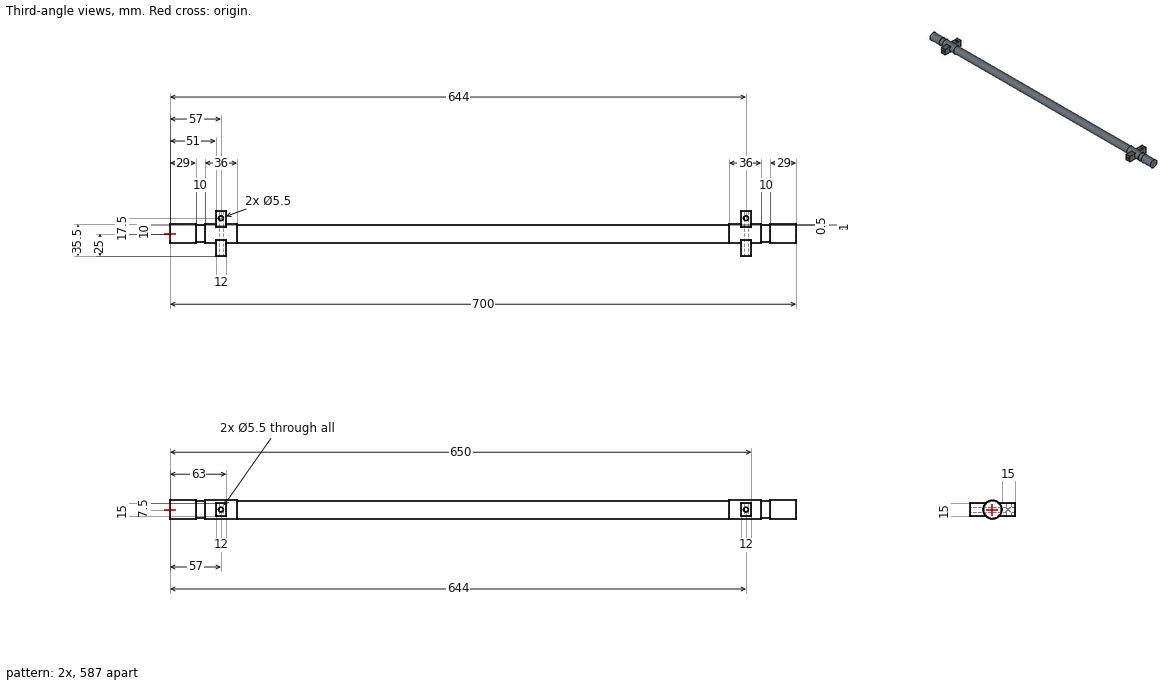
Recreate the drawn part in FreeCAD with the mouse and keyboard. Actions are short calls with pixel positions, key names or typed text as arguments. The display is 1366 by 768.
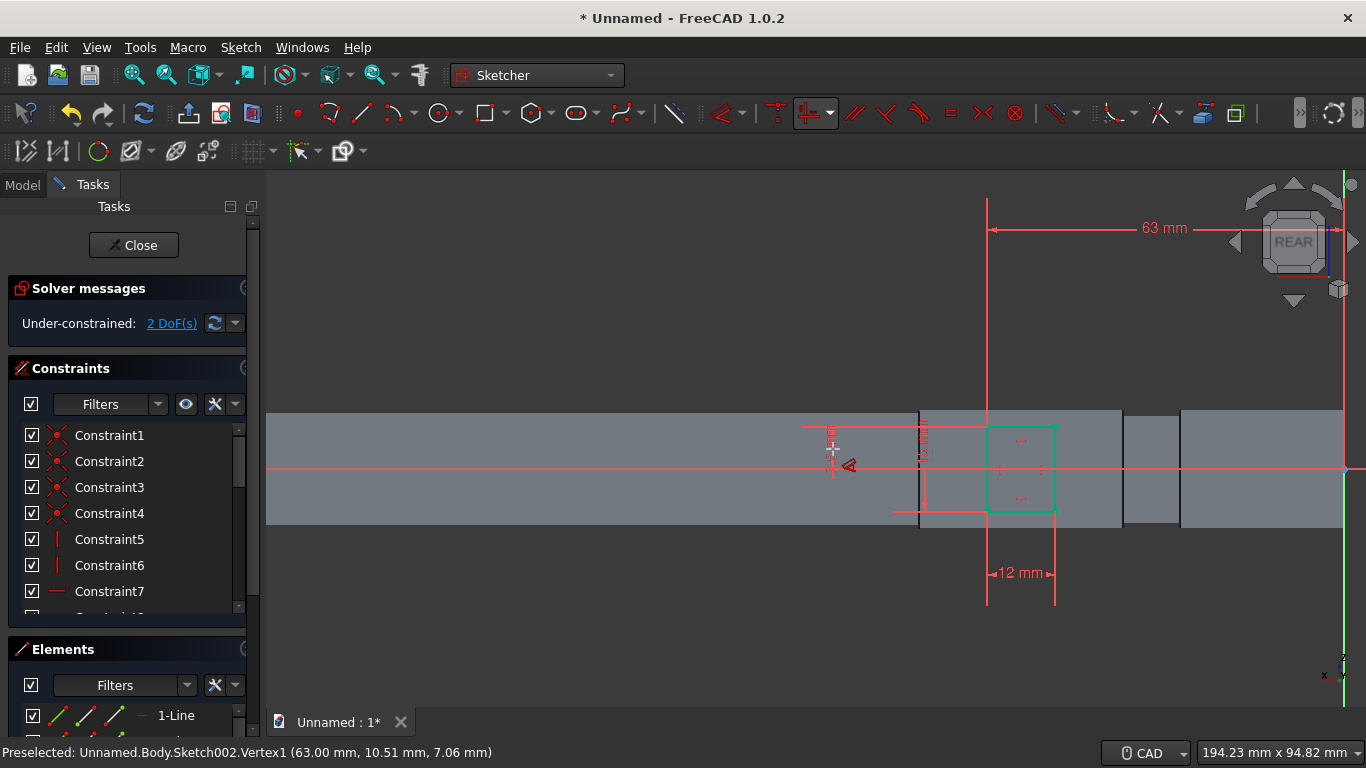
scroll(994, 432, down, 9)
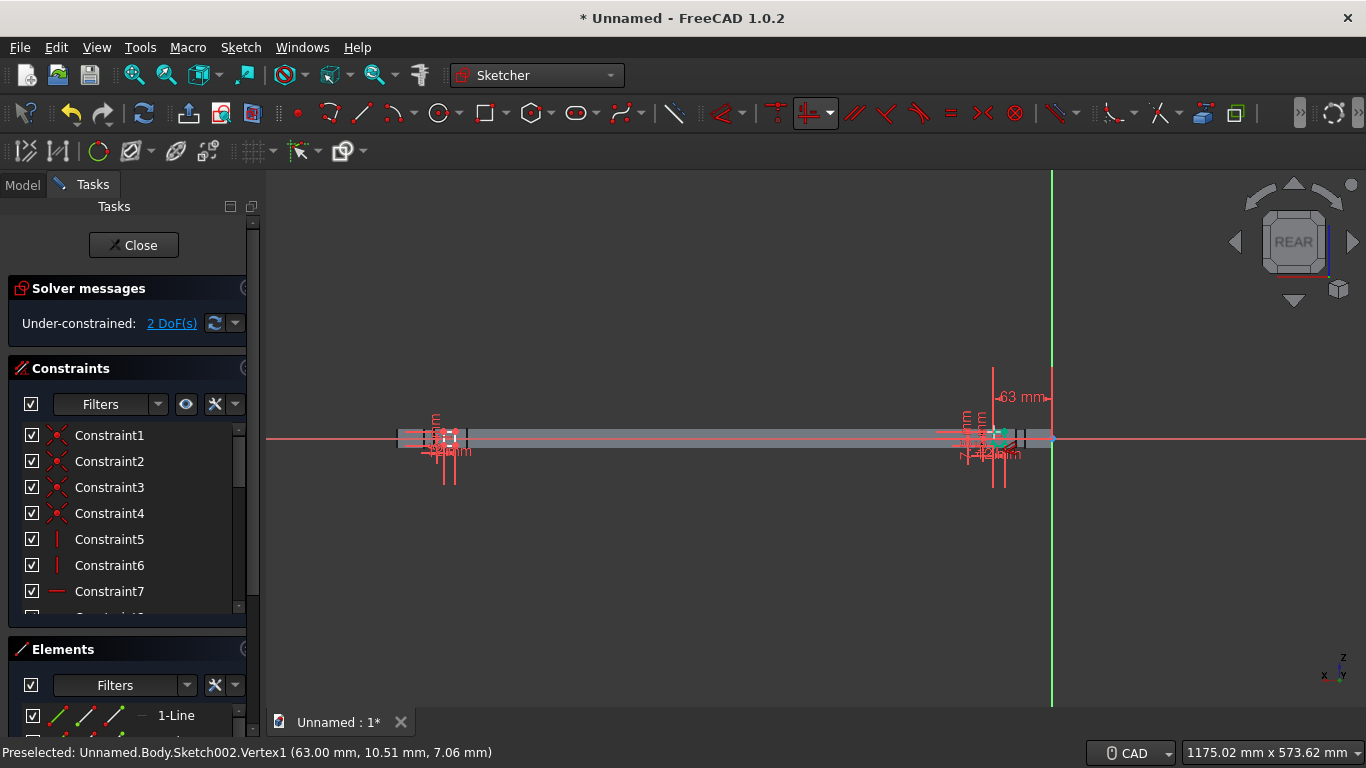
click(444, 432)
click(748, 398)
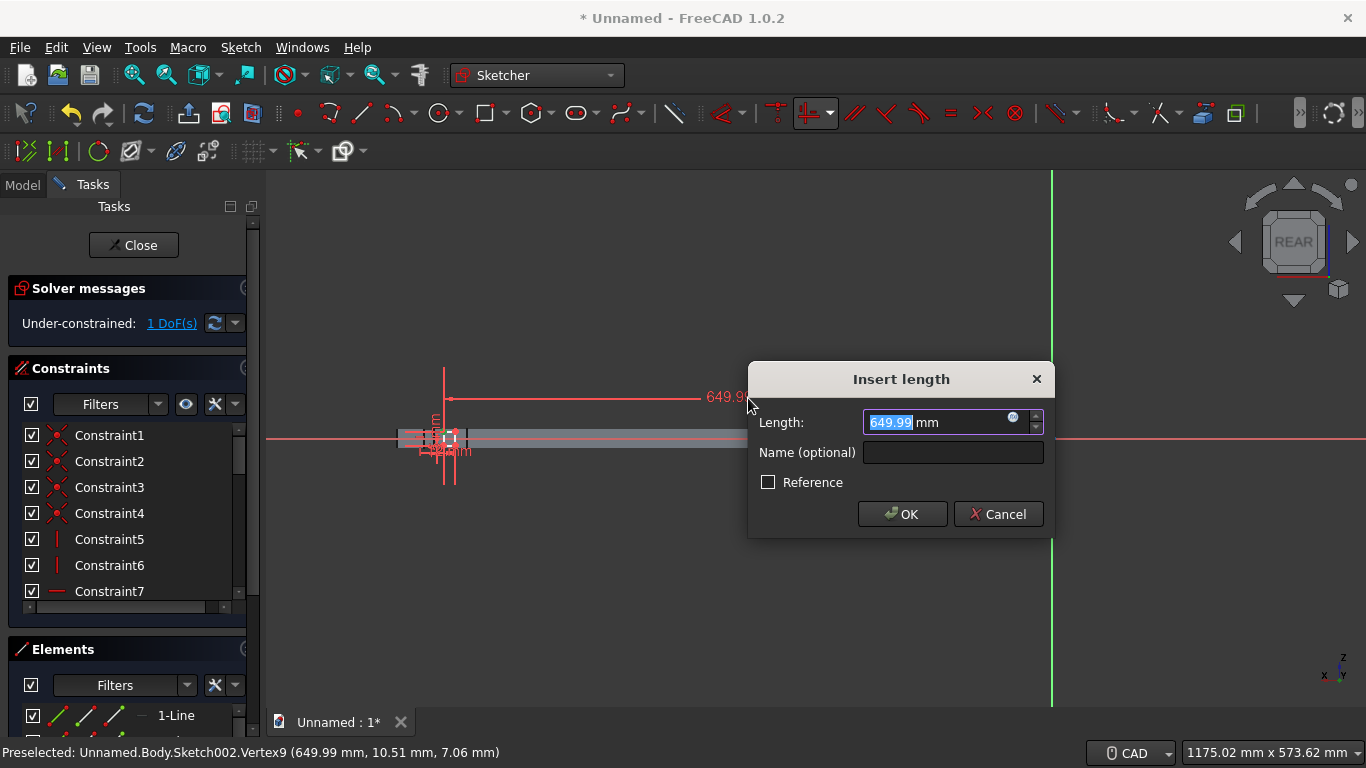
text(650)
key(Return)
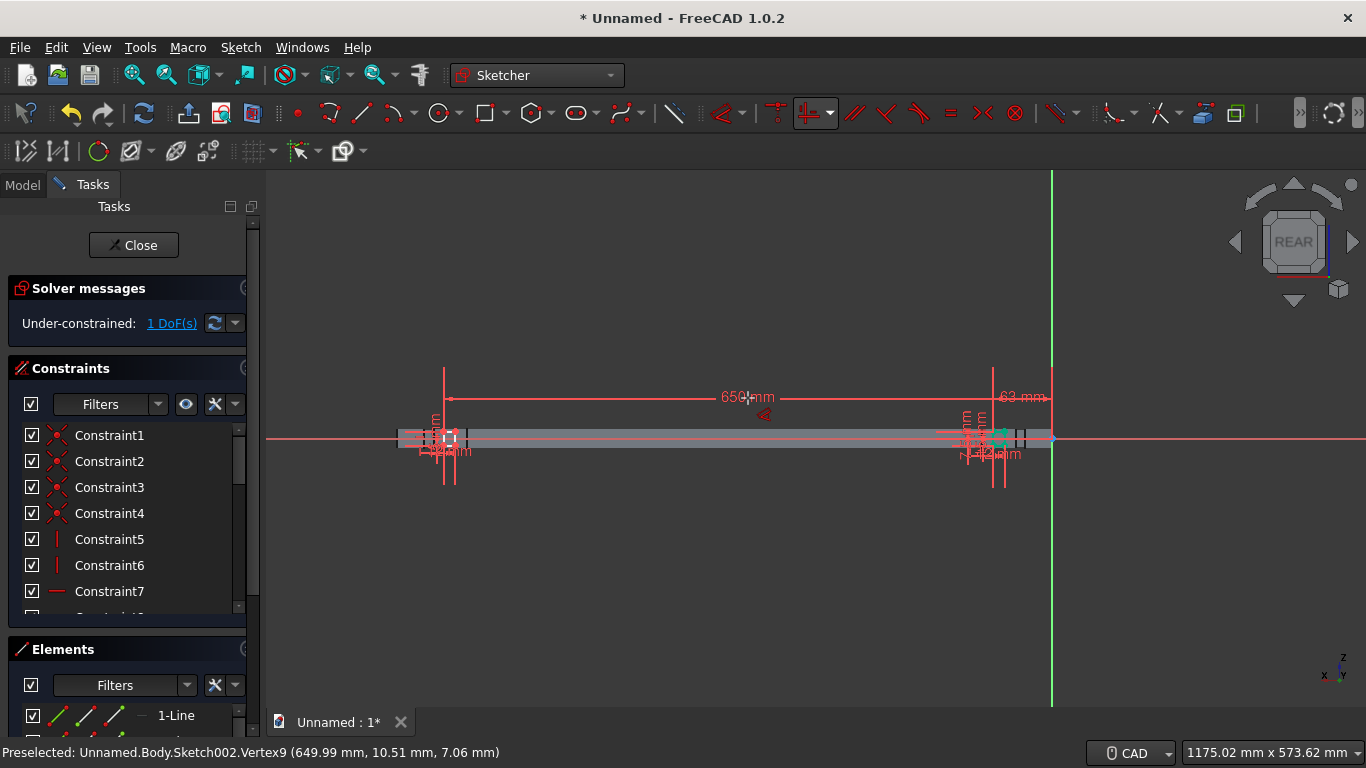
scroll(444, 432, up, 9)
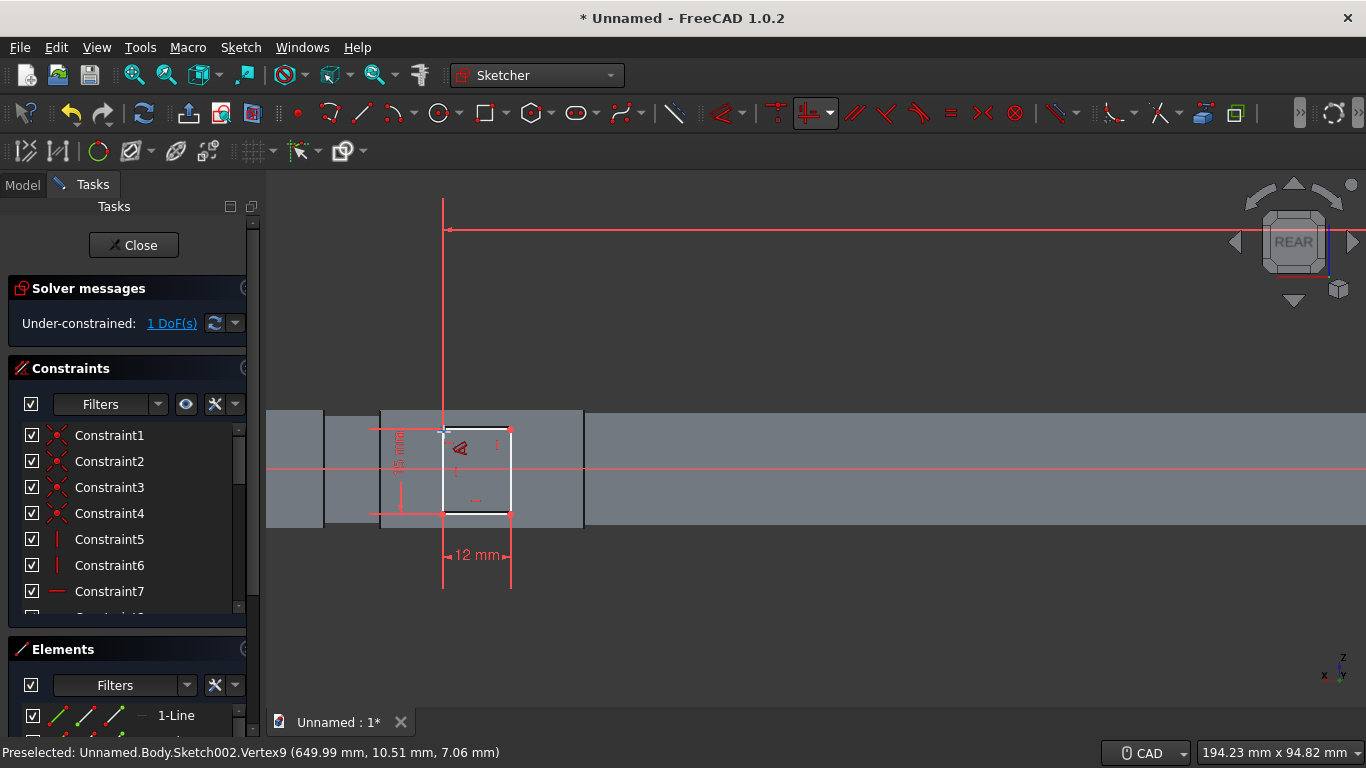
click(443, 429)
click(313, 449)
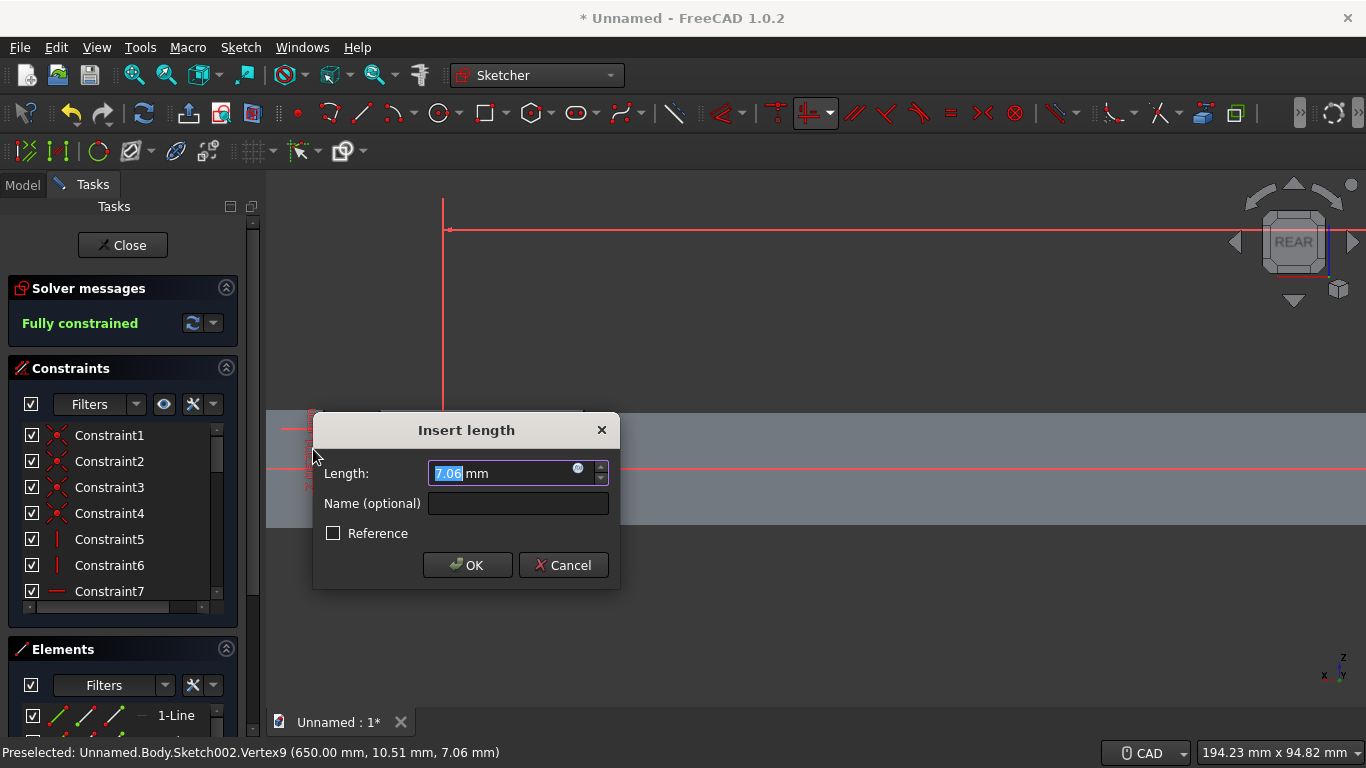
text(7.5)
key(Return)
key(Escape)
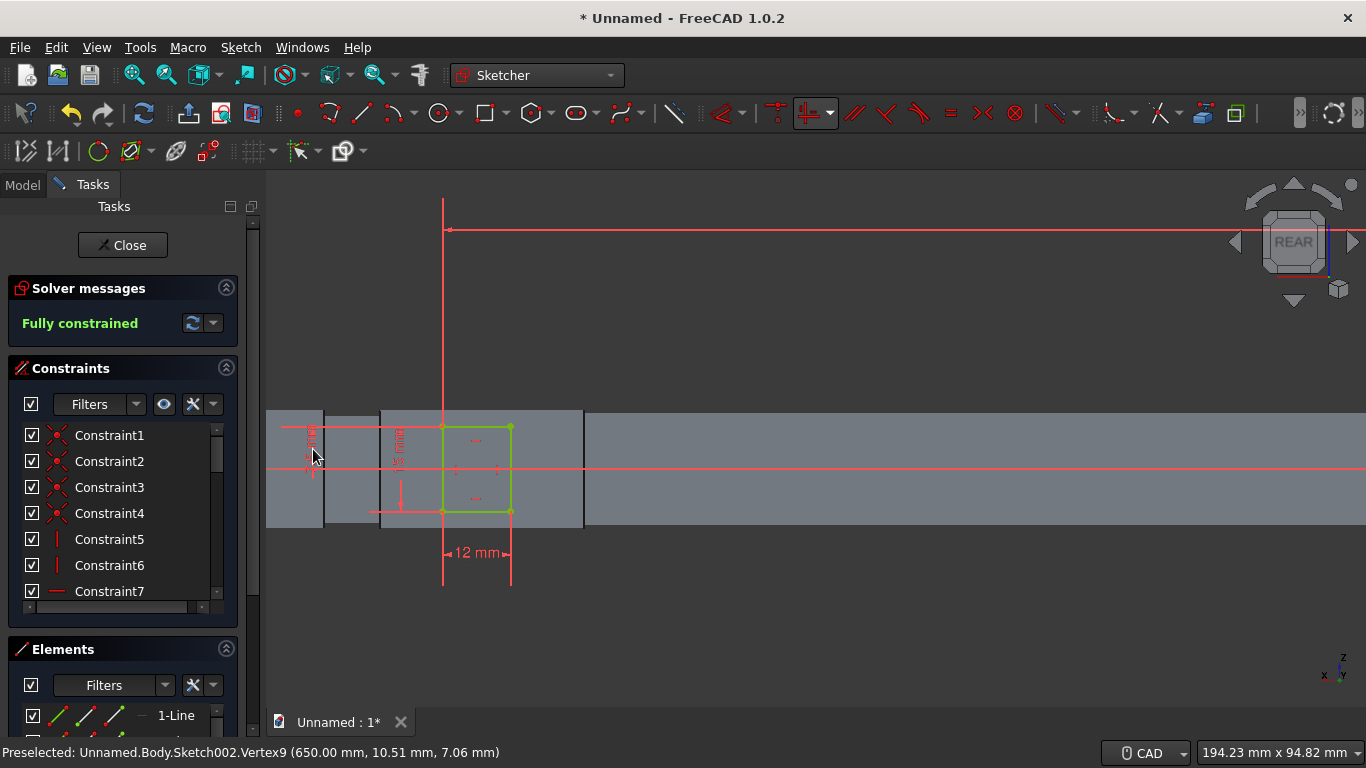
click(123, 245)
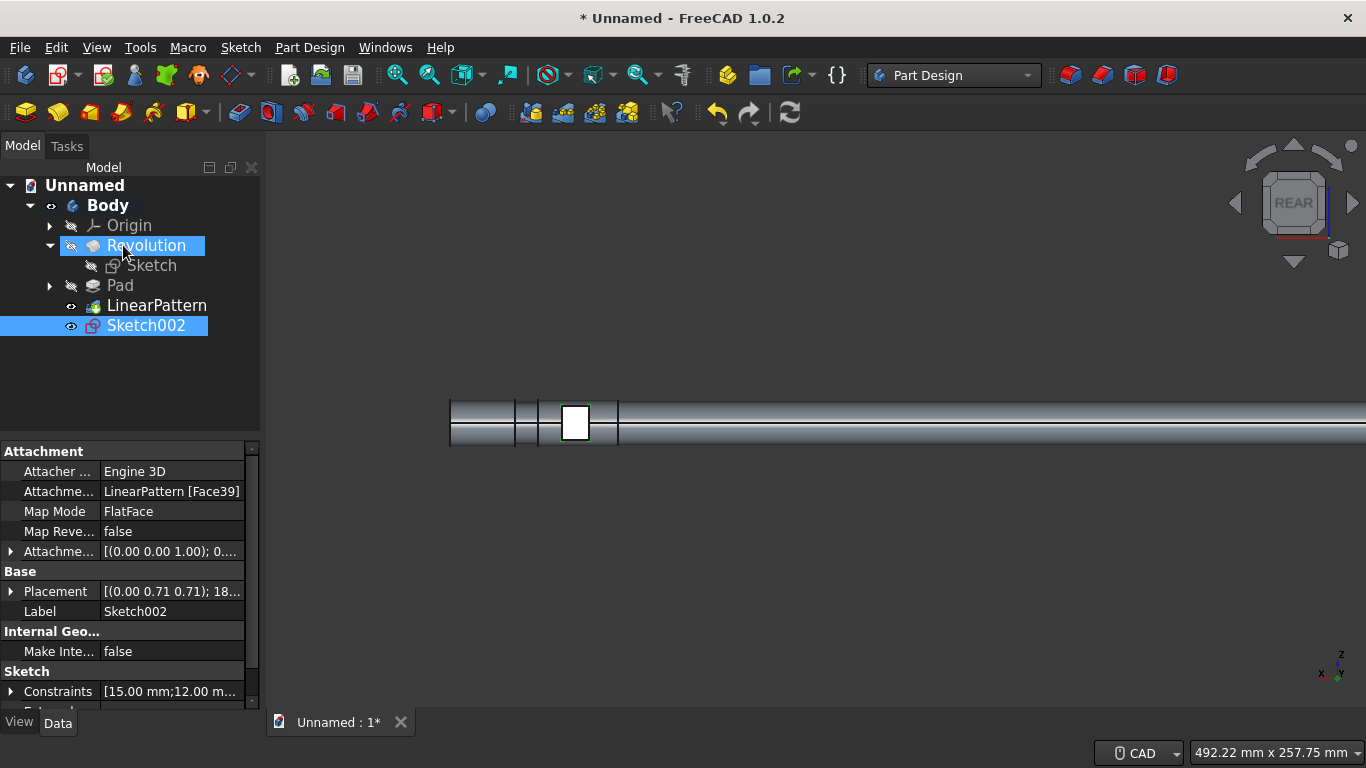
click(26, 112)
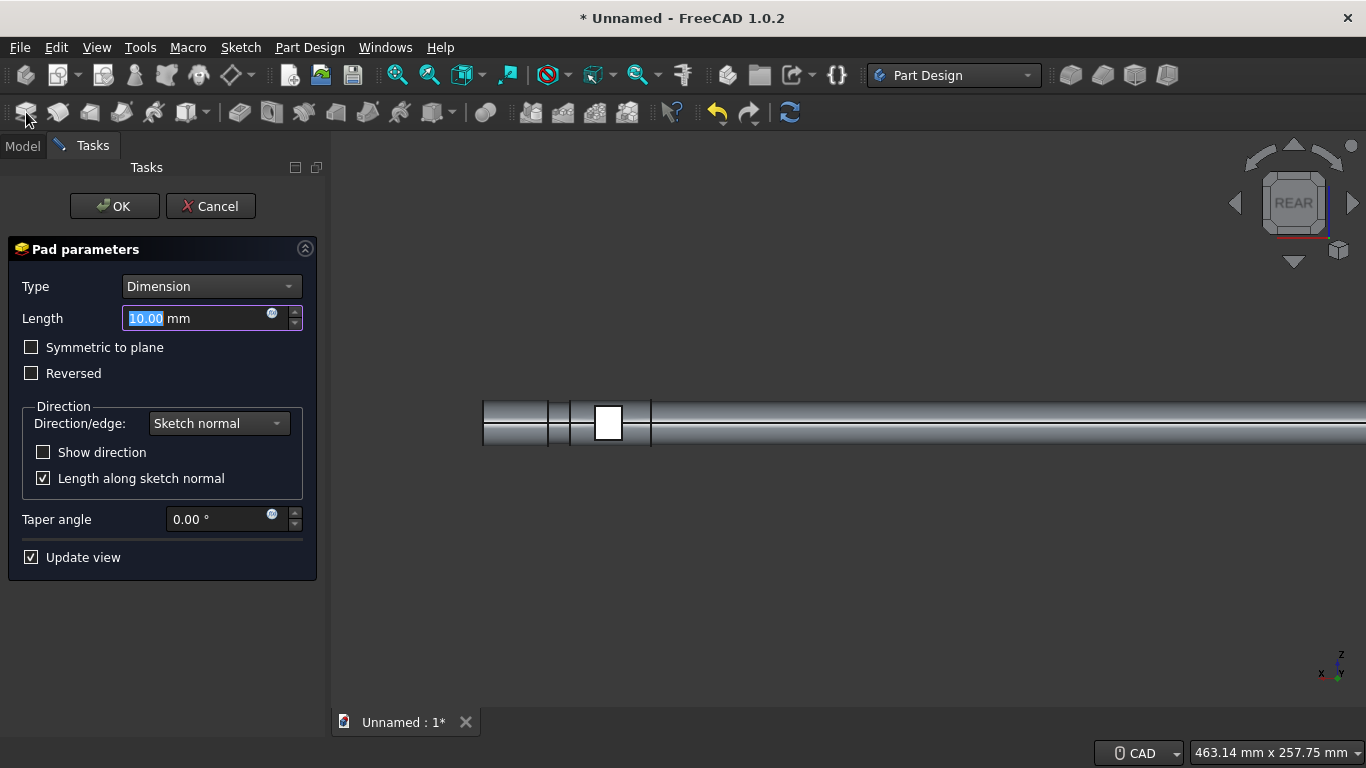
text(15)
key(Tab)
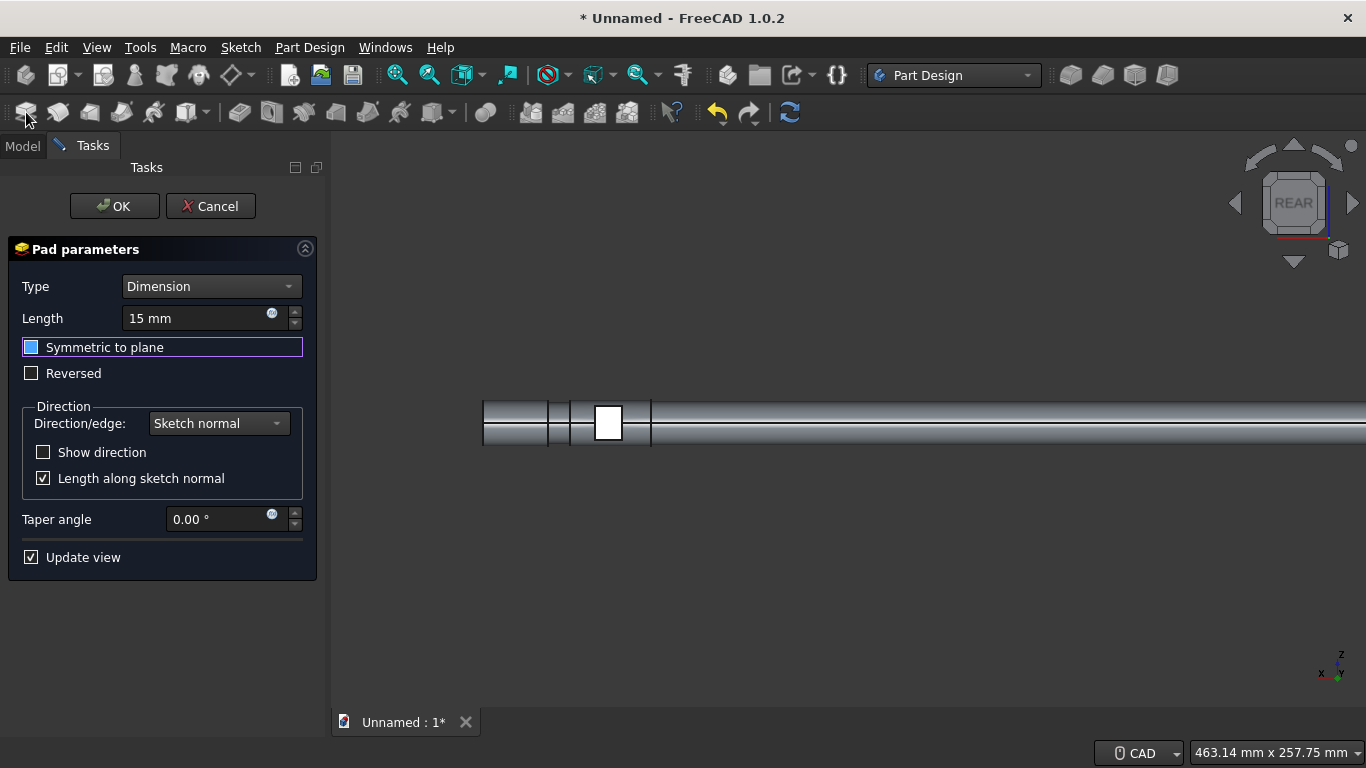
click(115, 206)